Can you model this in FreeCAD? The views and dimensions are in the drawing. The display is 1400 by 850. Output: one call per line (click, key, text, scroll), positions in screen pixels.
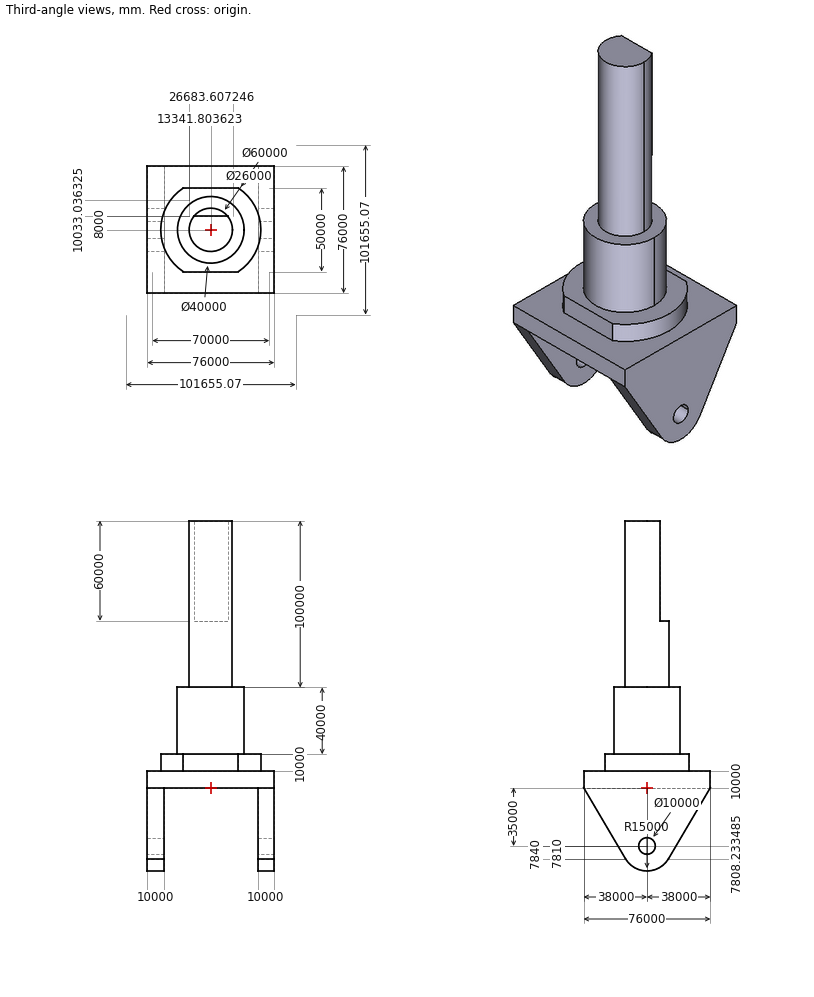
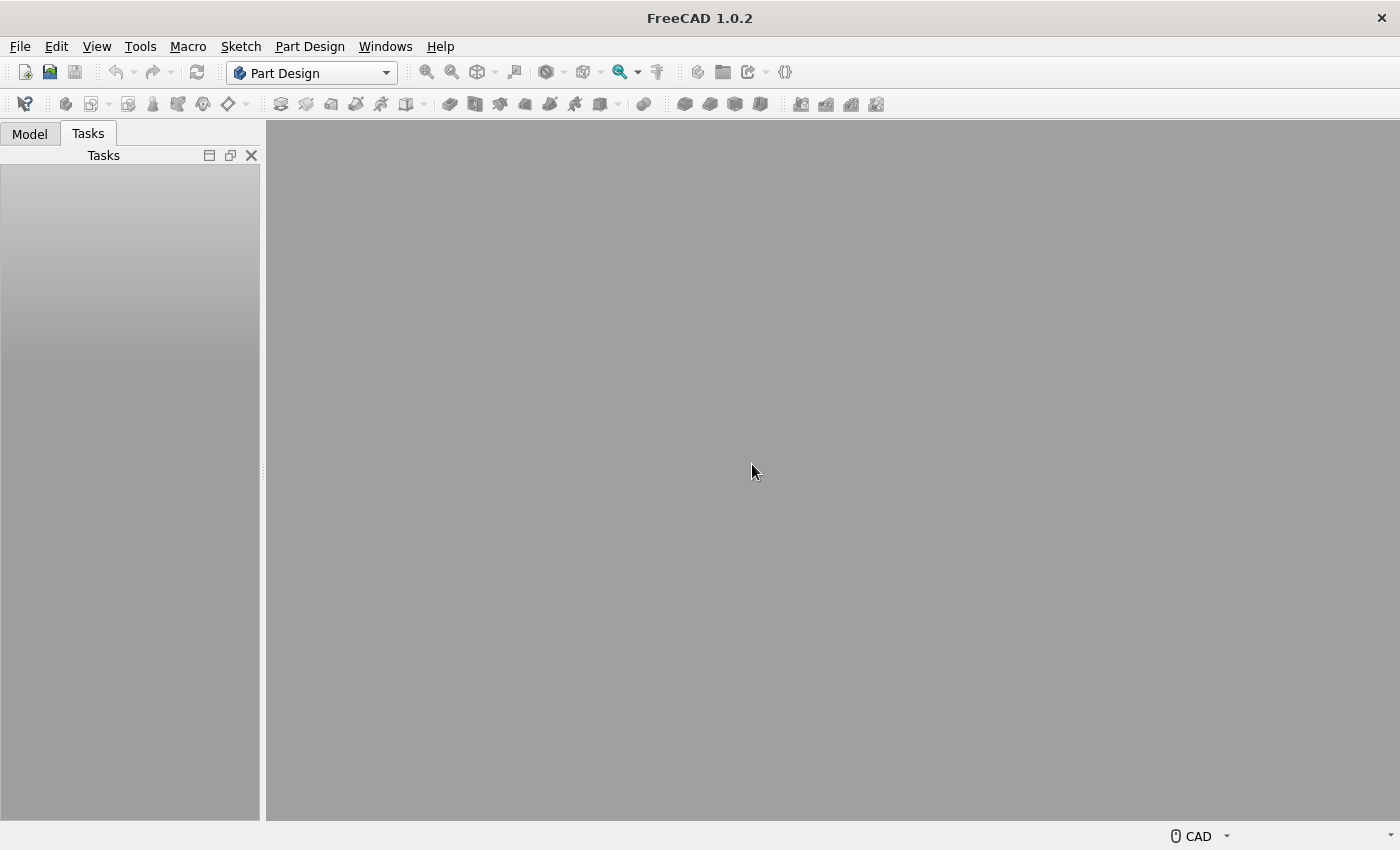
click(25, 72)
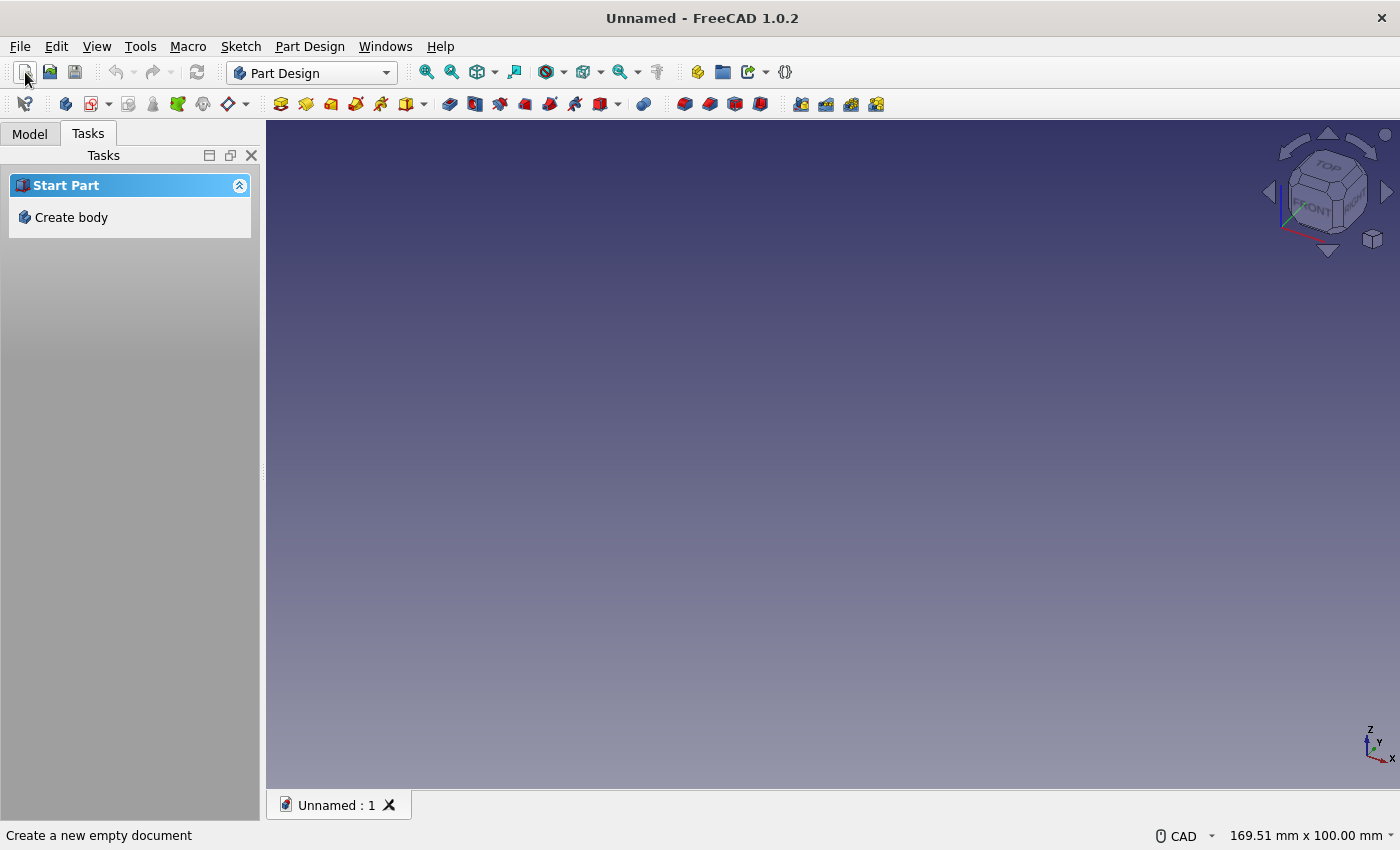
click(90, 104)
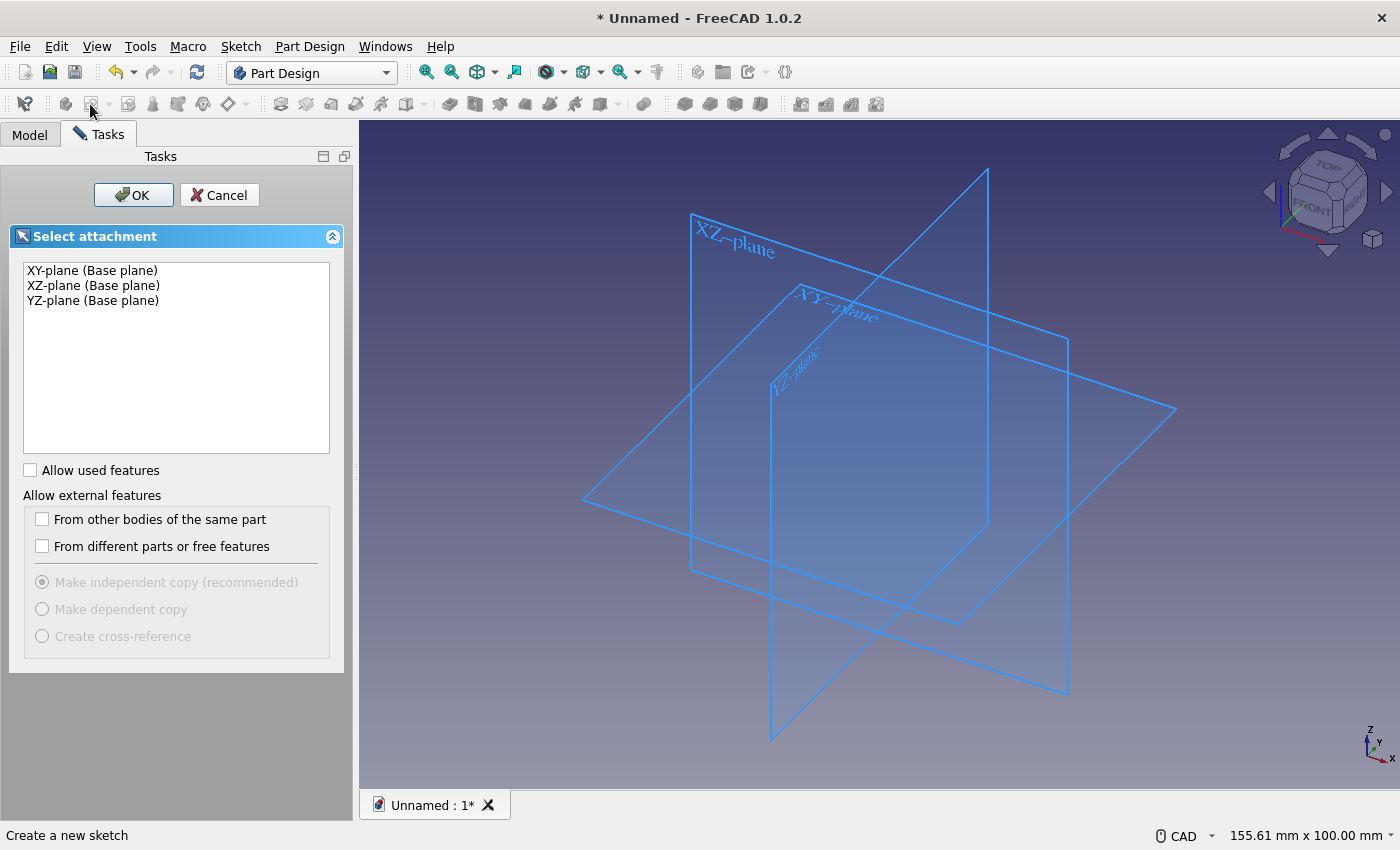
click(84, 270)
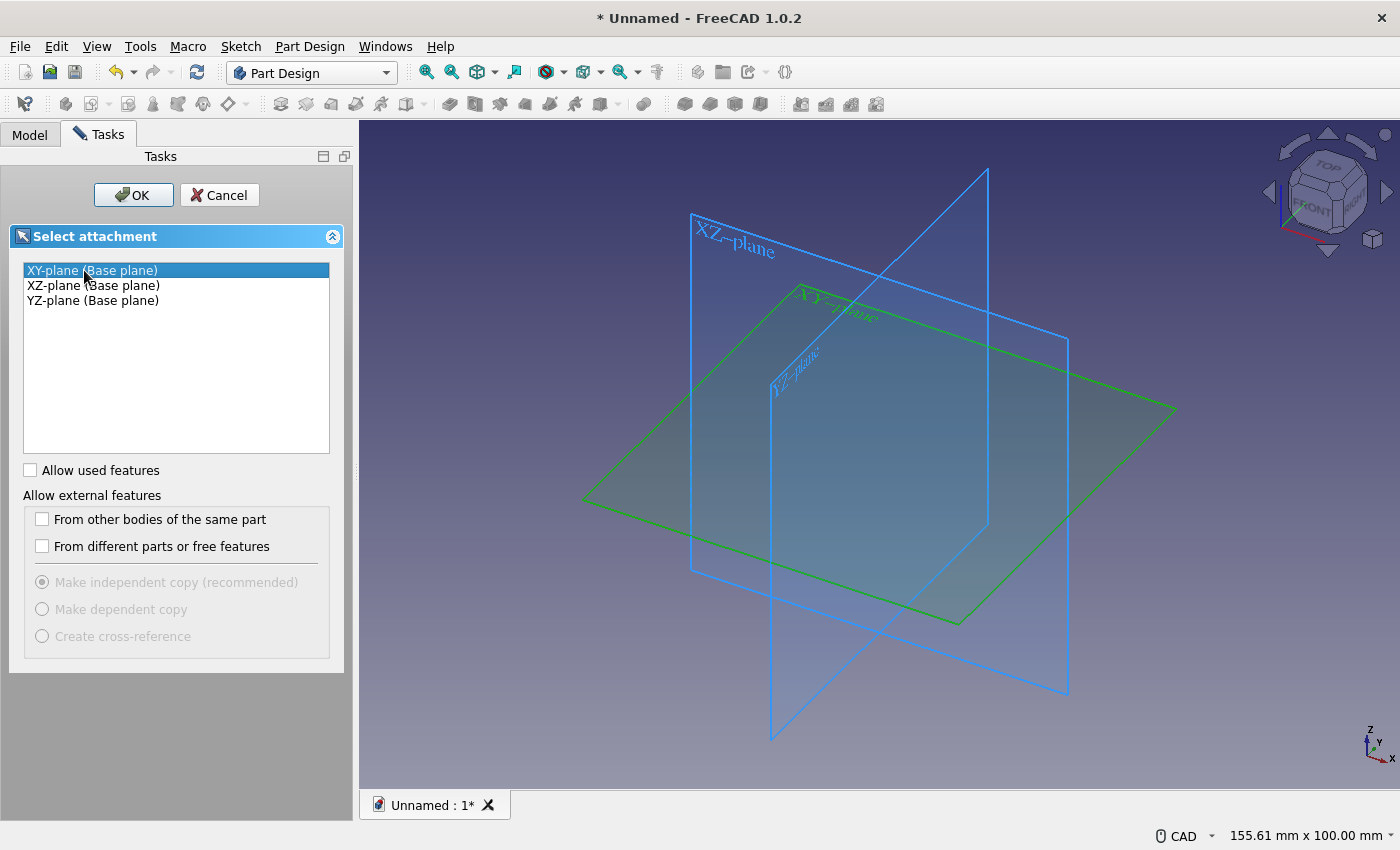
click(134, 195)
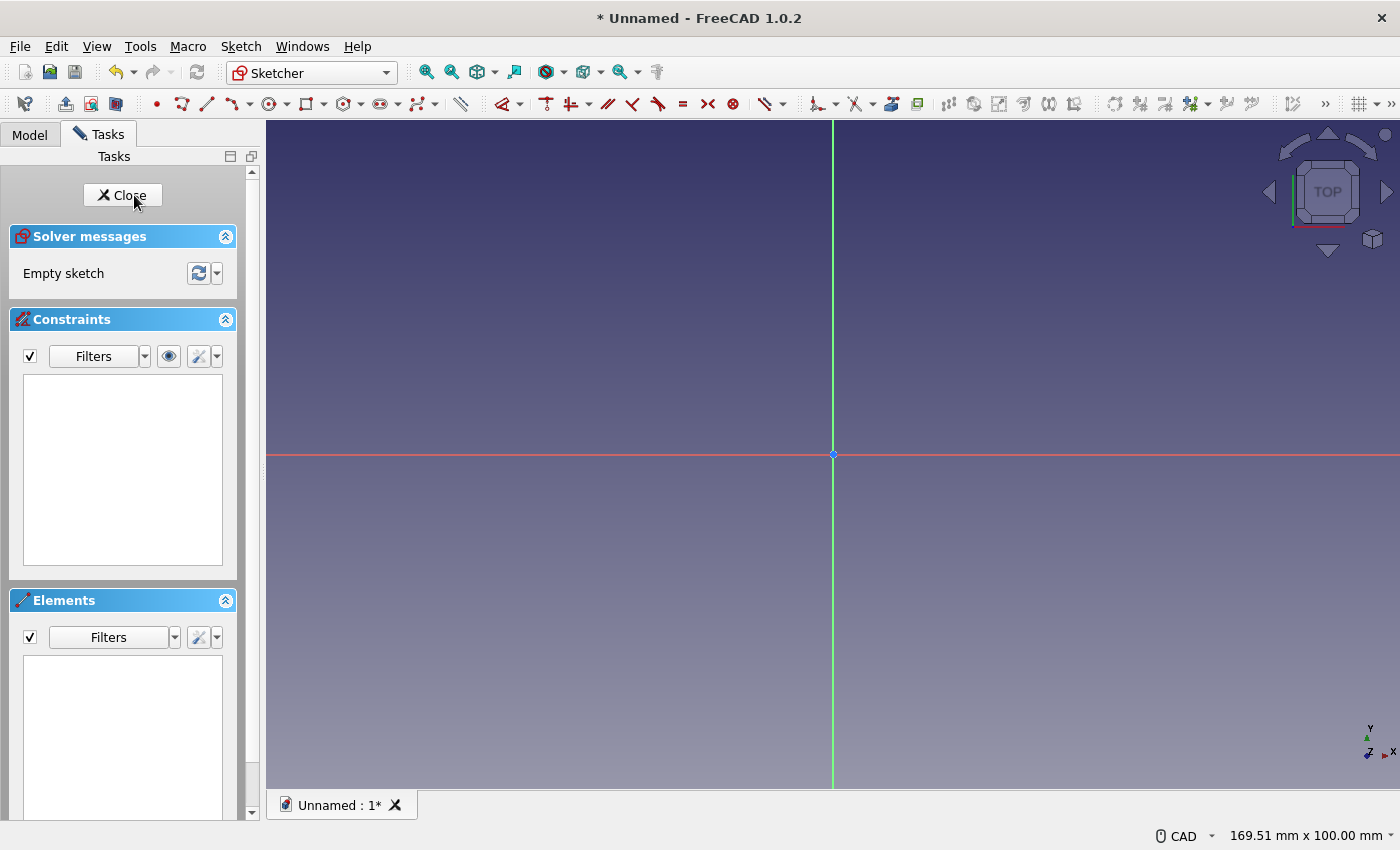
scroll(764, 454, down, 15)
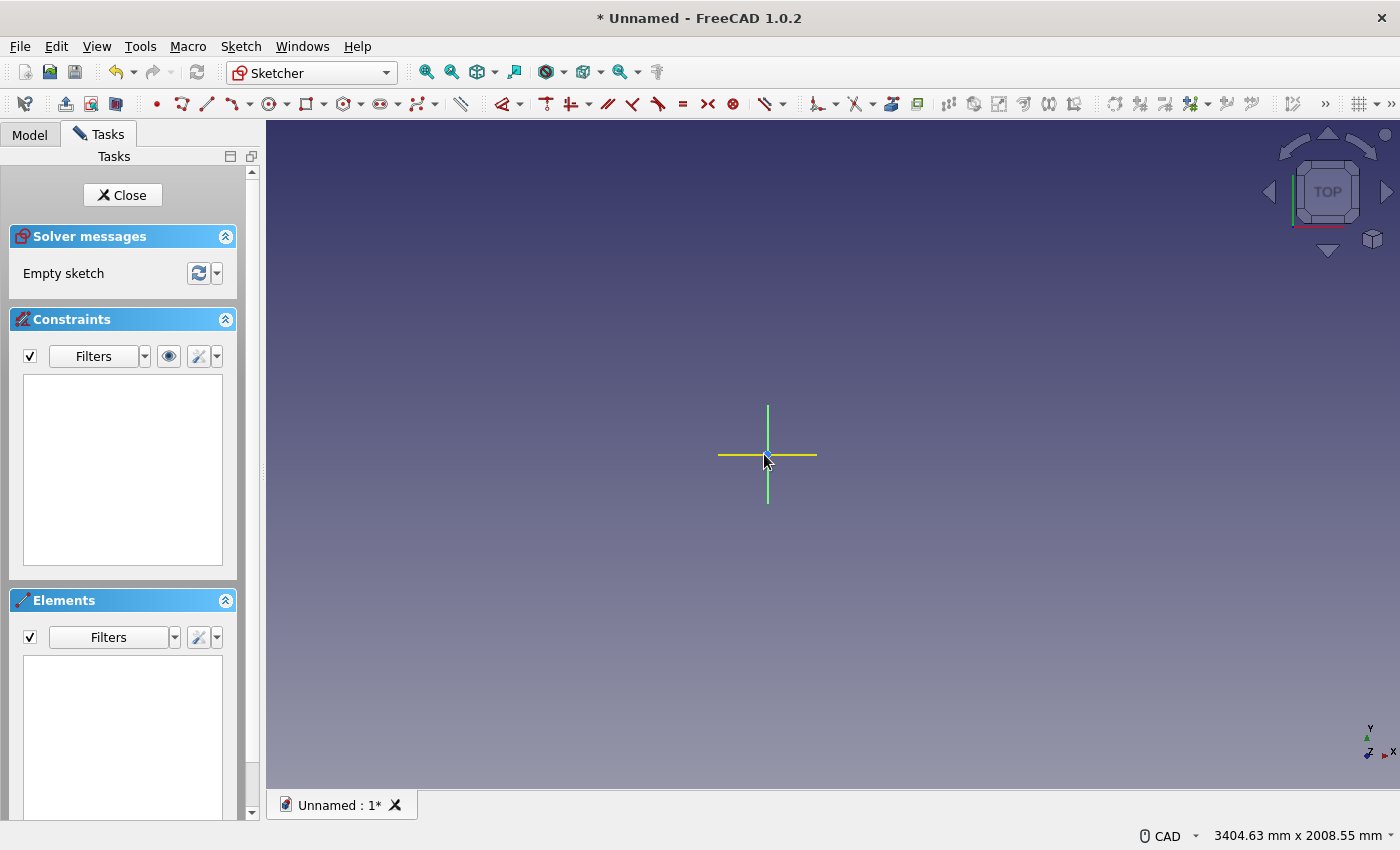
scroll(764, 454, down, 15)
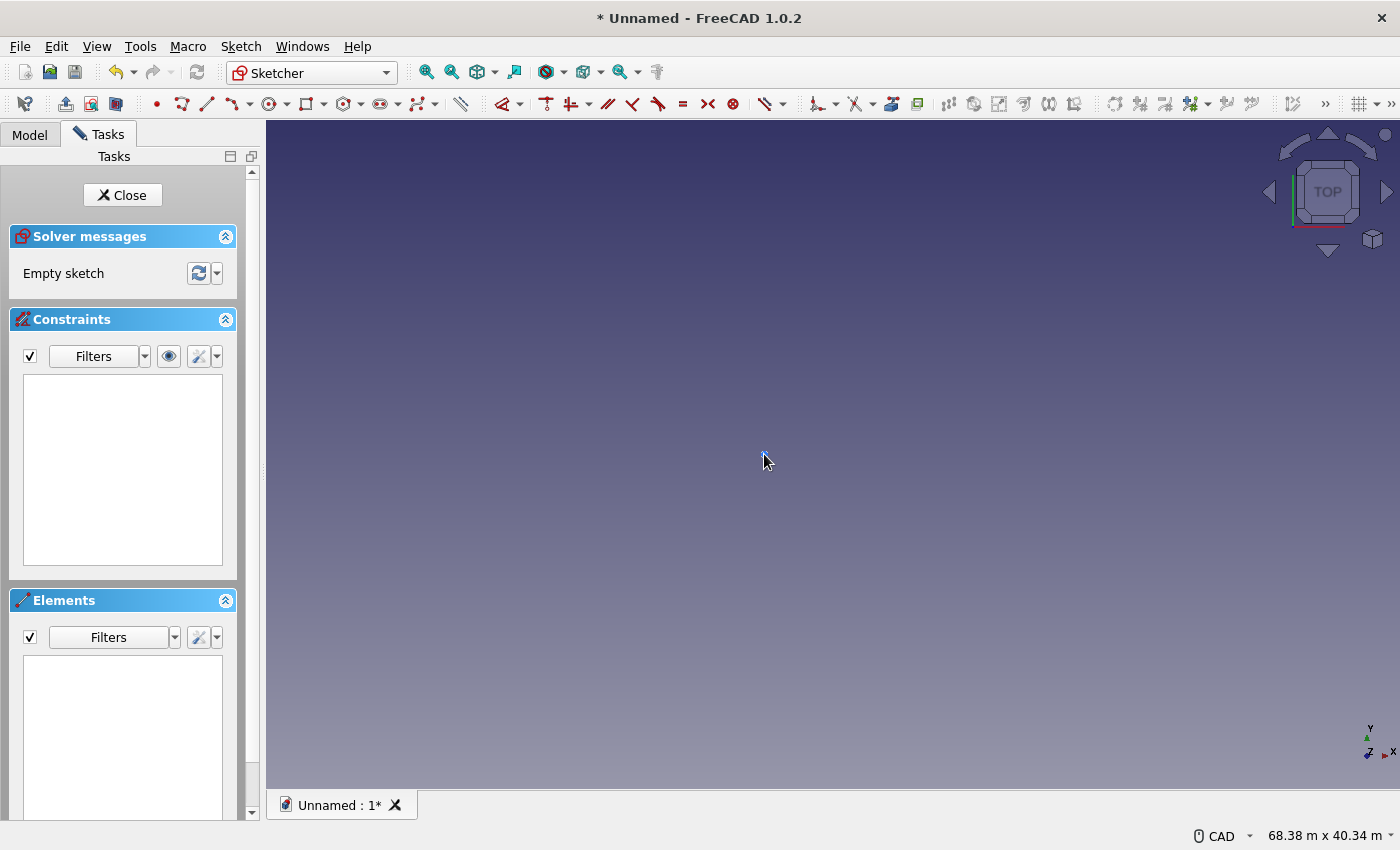
scroll(764, 454, down, 5)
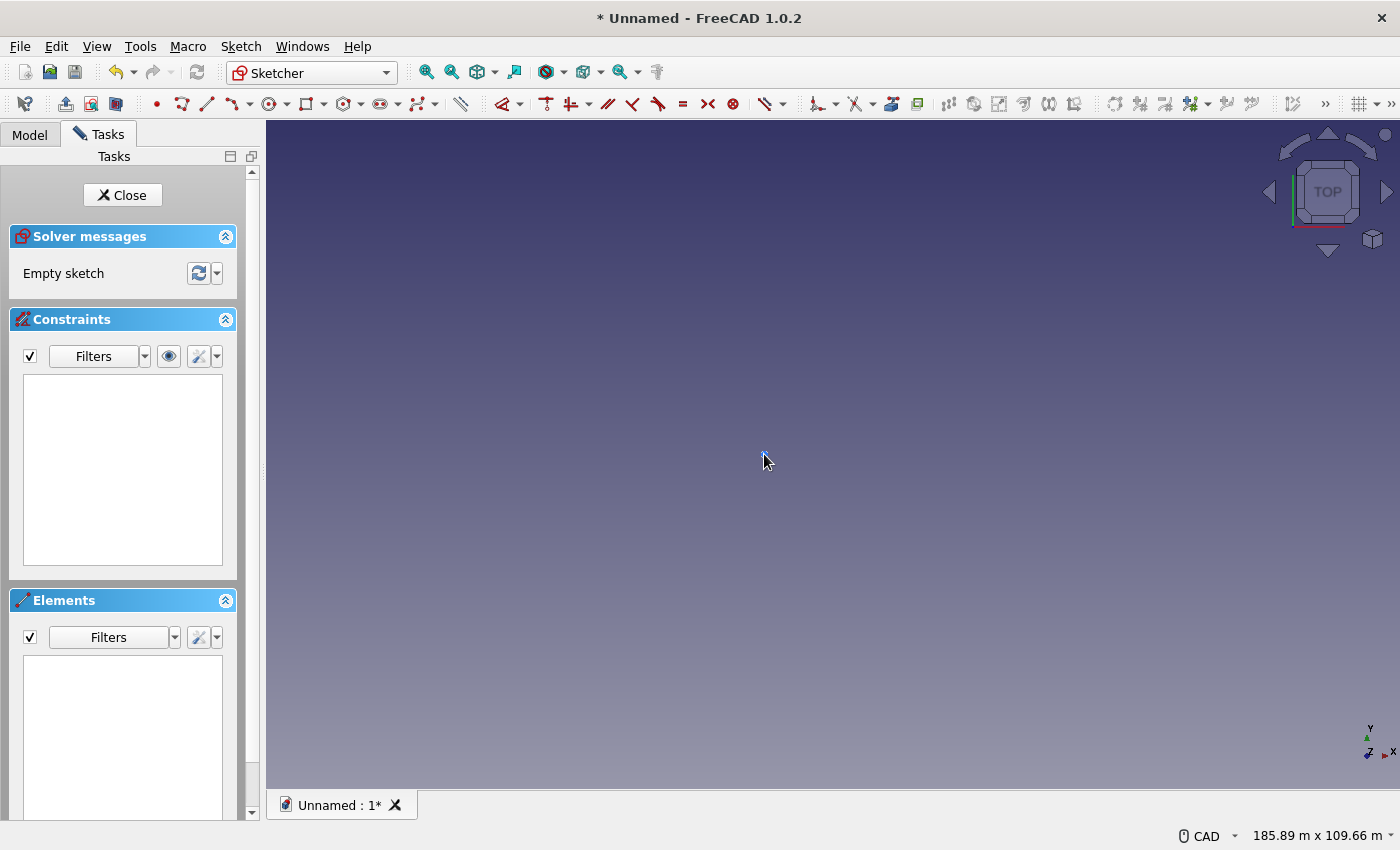
click(324, 104)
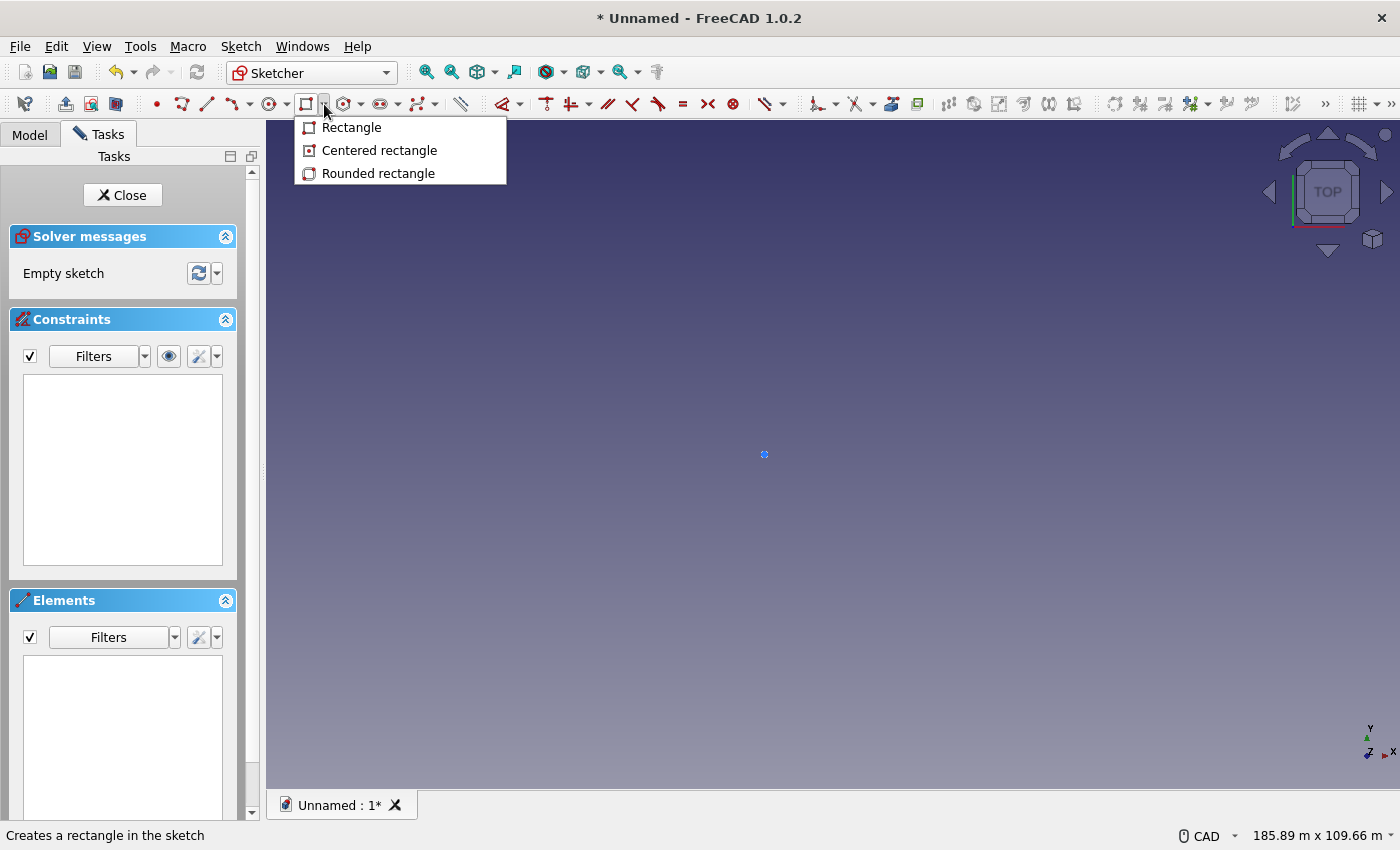
click(400, 150)